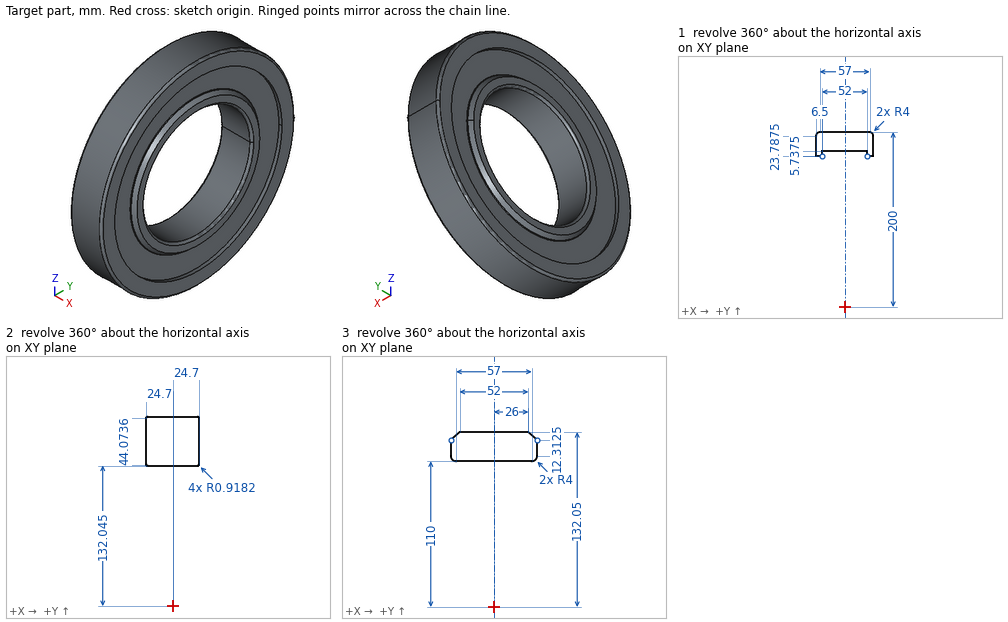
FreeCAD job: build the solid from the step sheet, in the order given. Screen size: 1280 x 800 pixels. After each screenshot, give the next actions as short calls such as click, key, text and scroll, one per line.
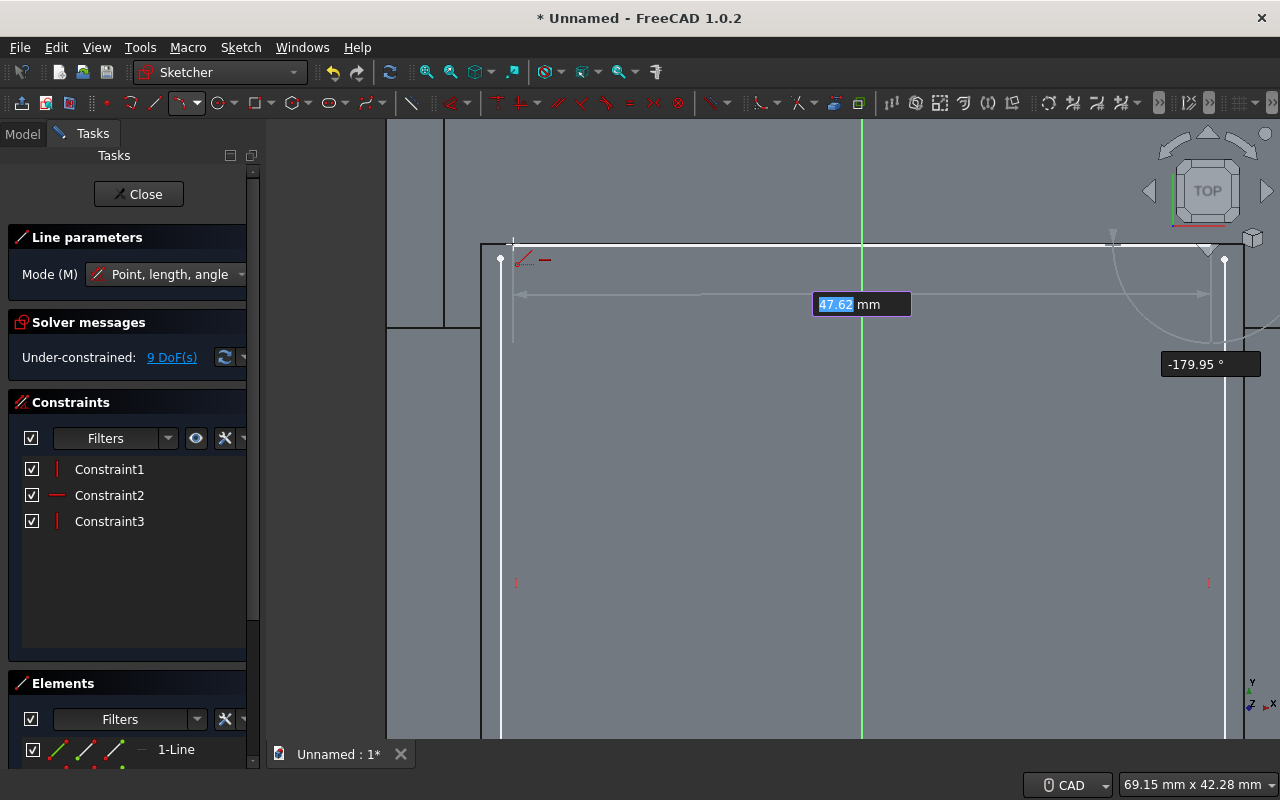
click(514, 244)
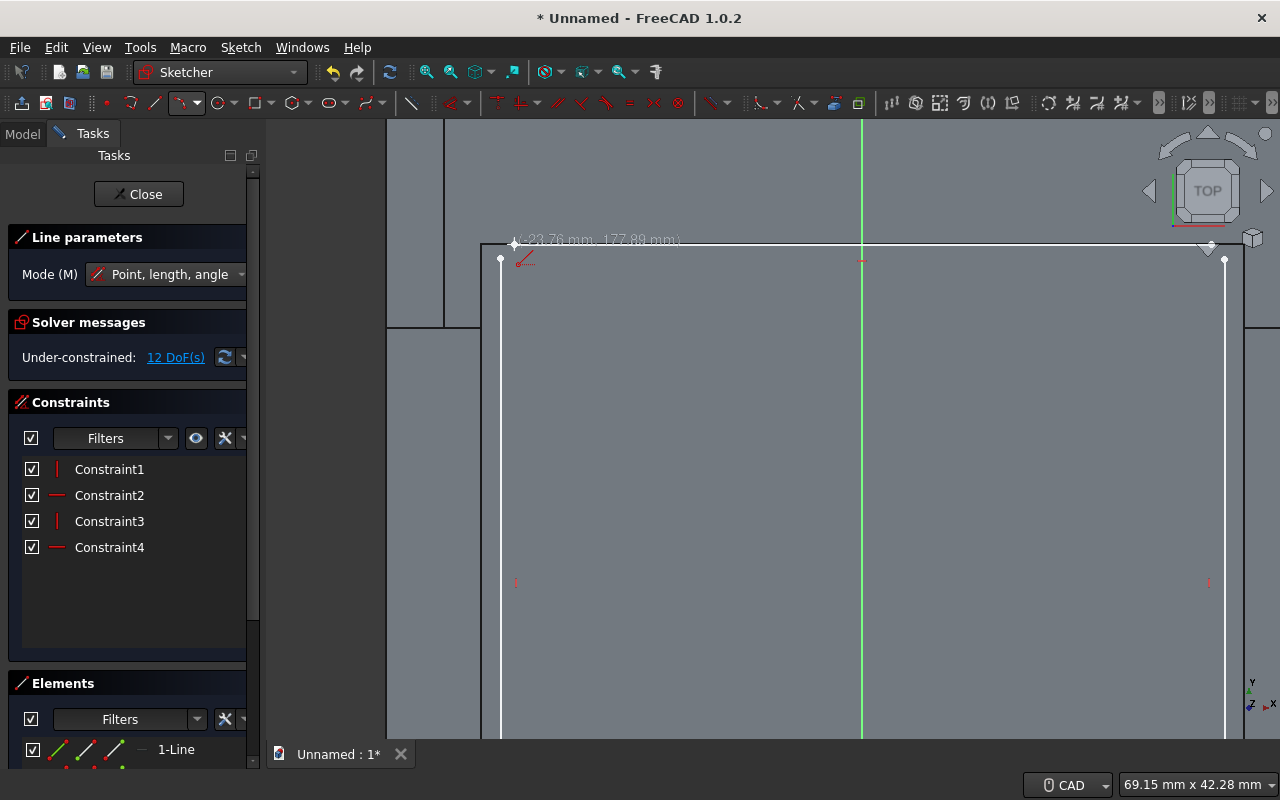
click(180, 104)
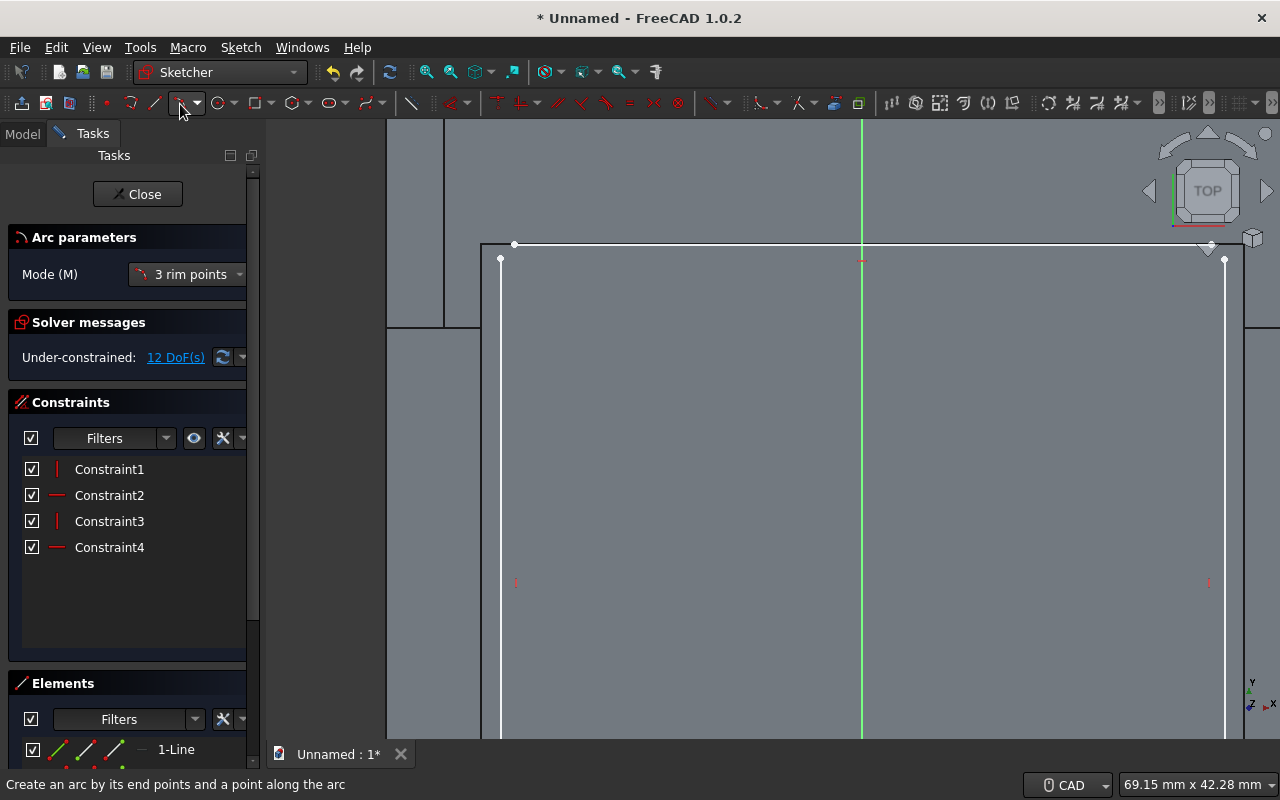
scroll(512, 244, down, 3)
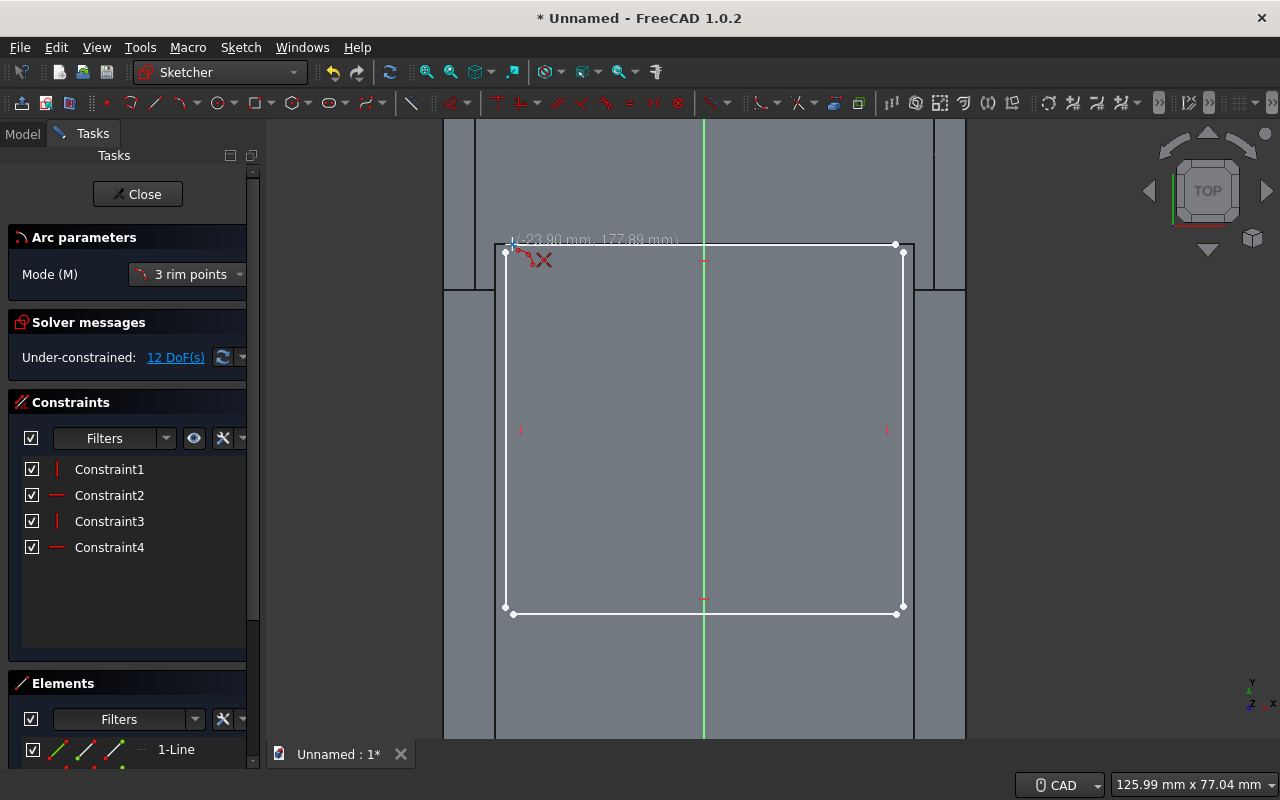
scroll(506, 606, up, 3)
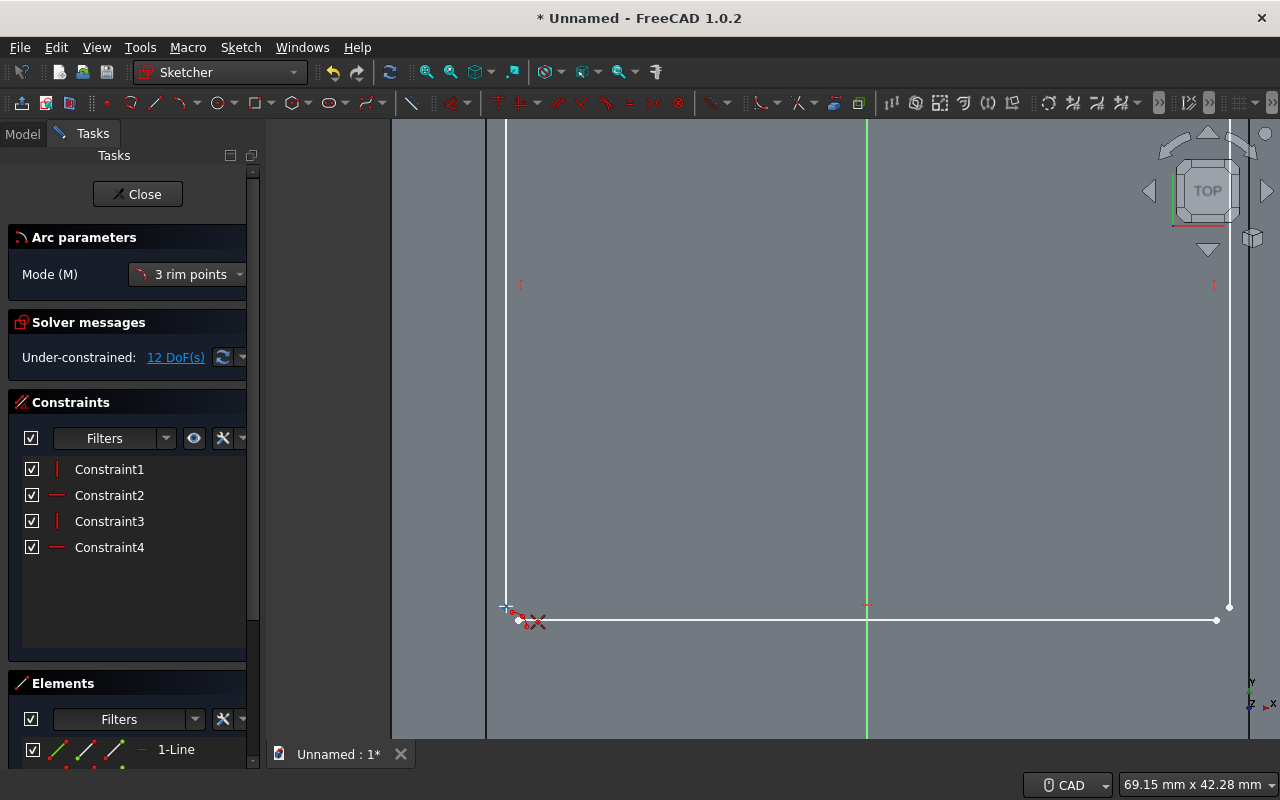
click(506, 608)
click(519, 620)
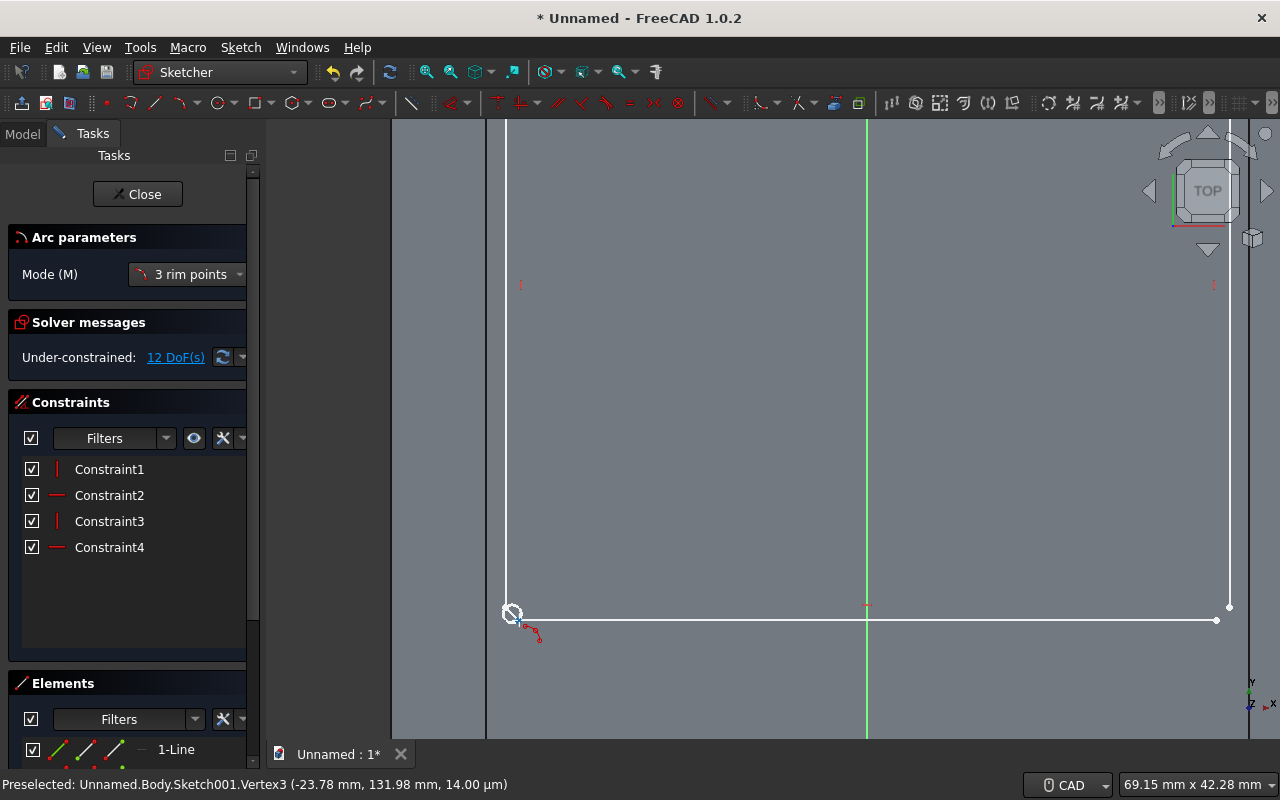
scroll(509, 615, up, 7)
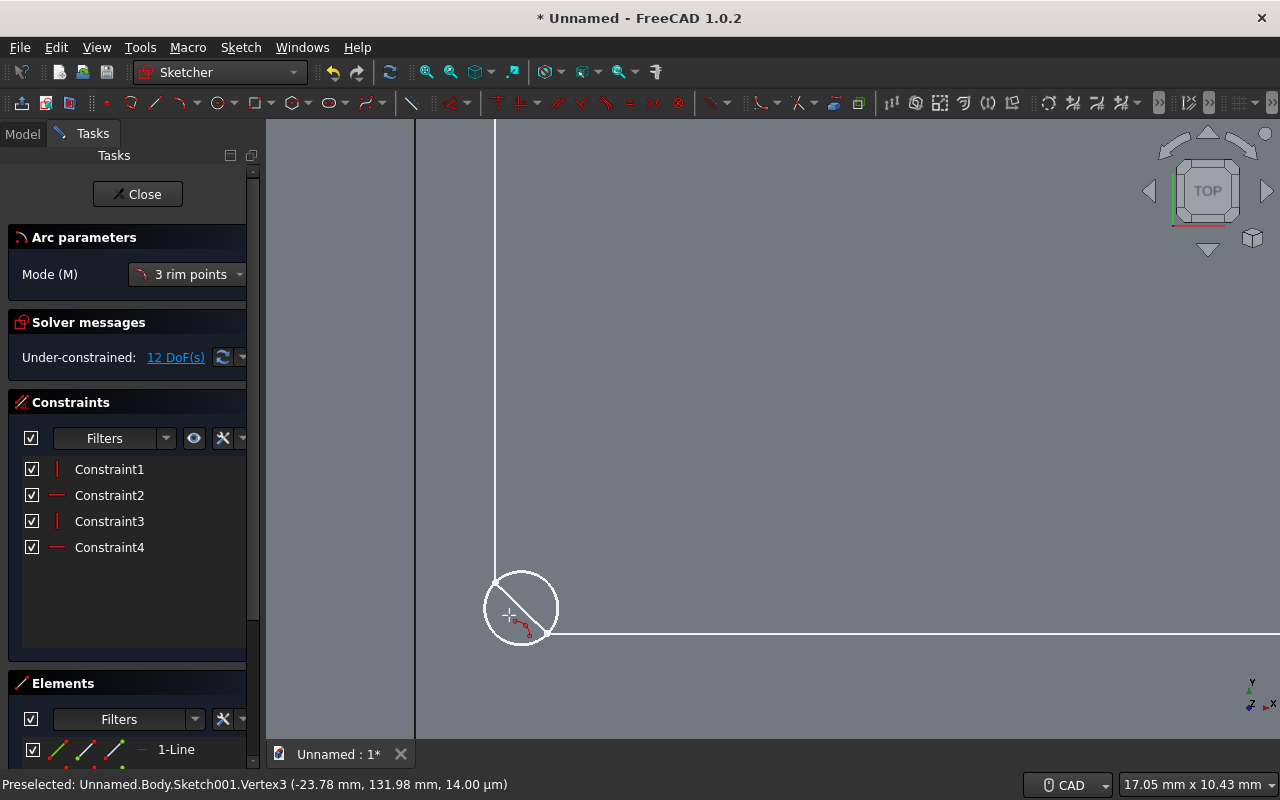
click(509, 614)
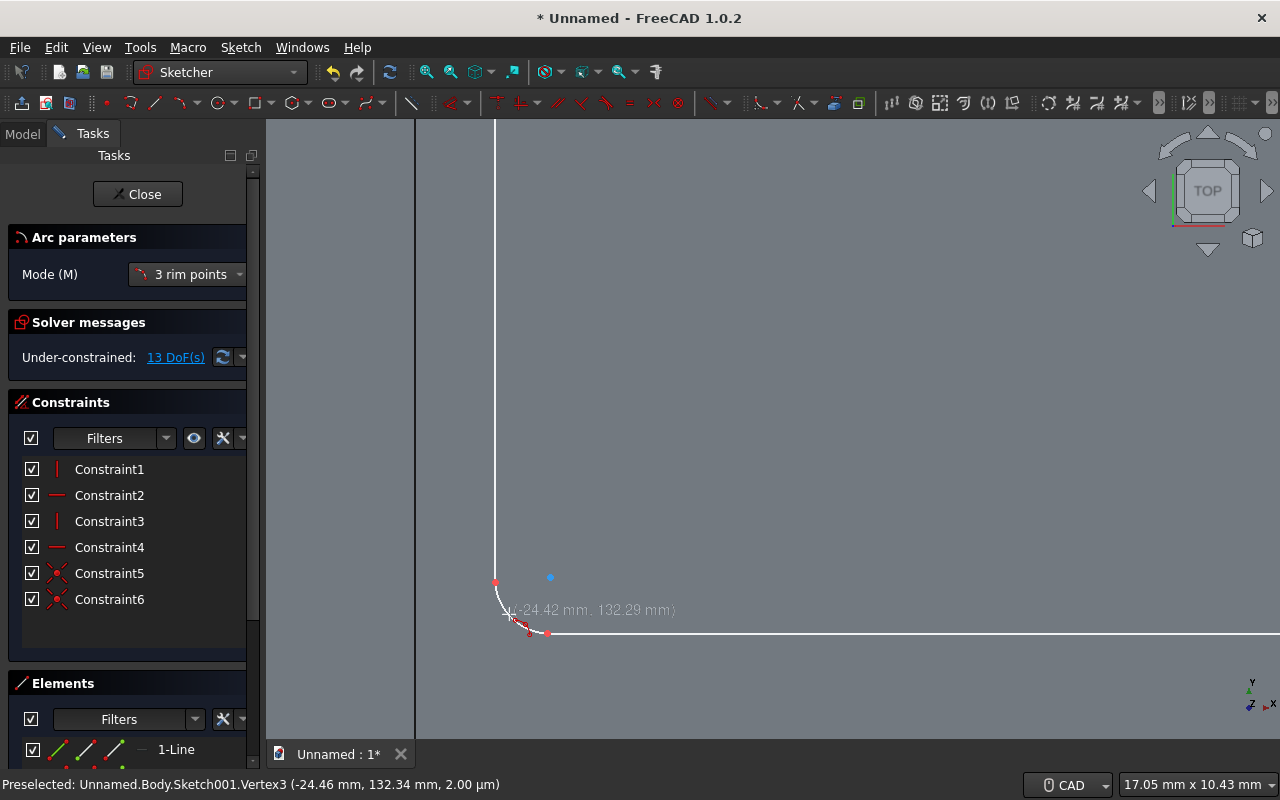
scroll(508, 611, down, 10)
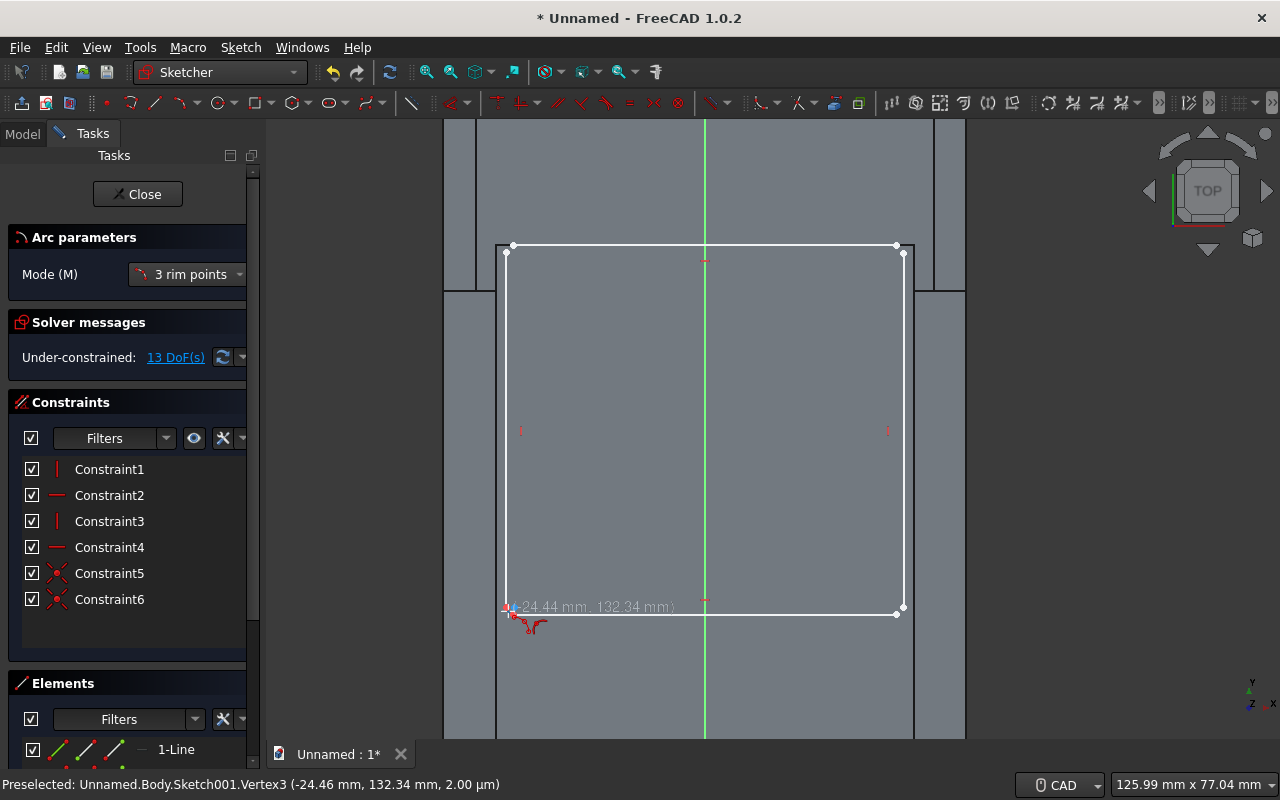
scroll(896, 614, up, 3)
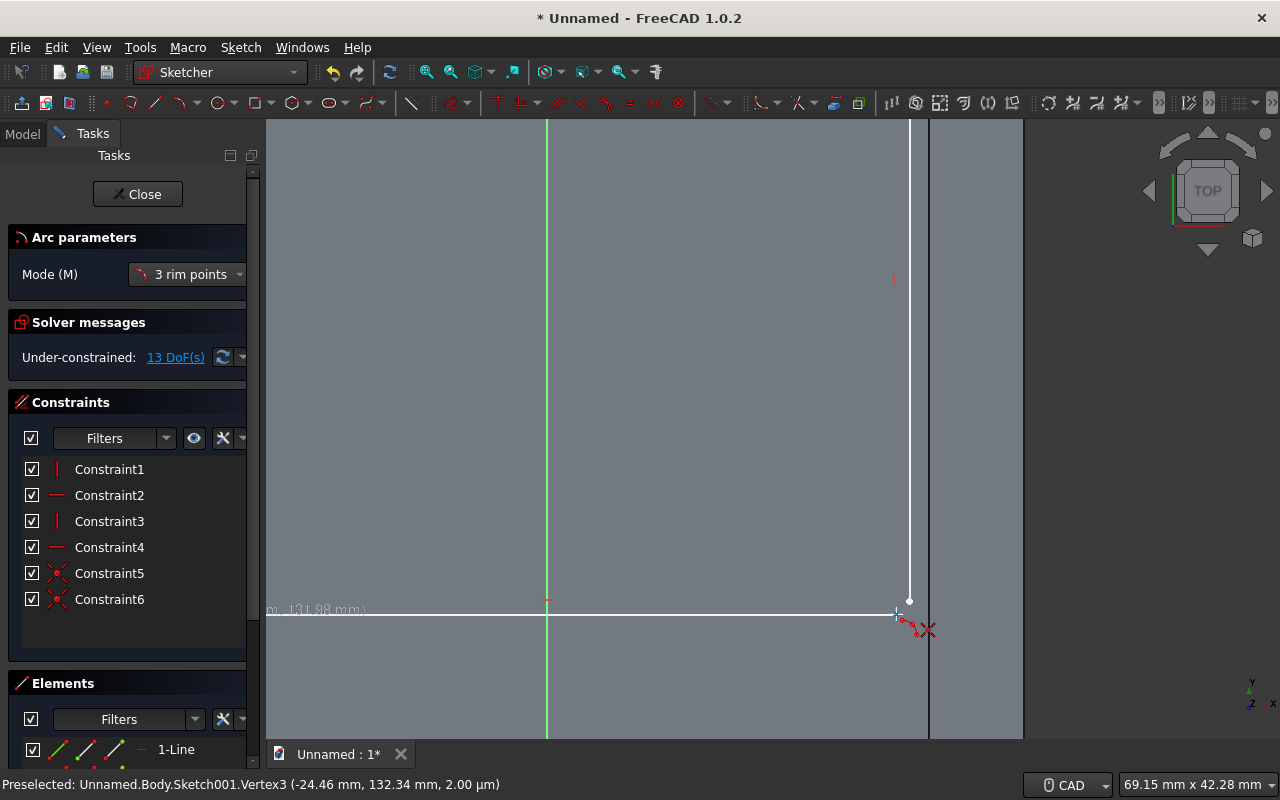
click(896, 615)
click(910, 602)